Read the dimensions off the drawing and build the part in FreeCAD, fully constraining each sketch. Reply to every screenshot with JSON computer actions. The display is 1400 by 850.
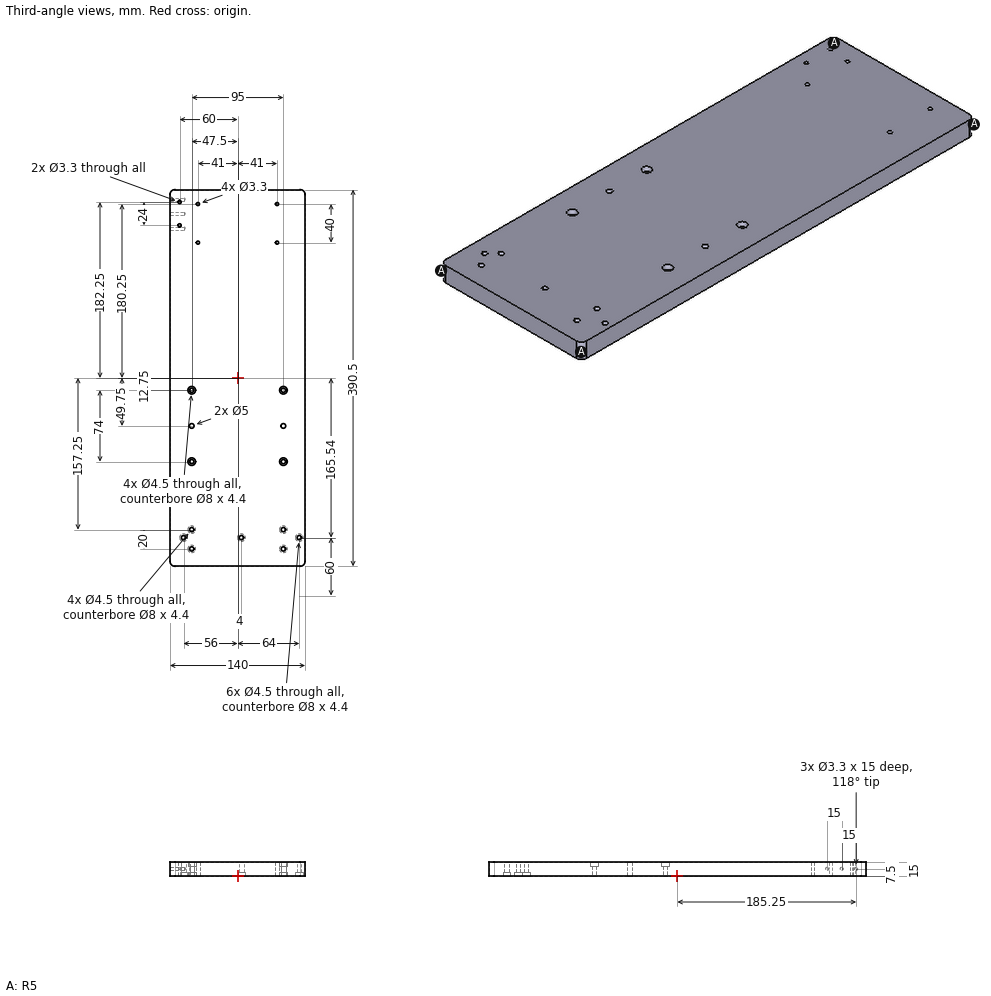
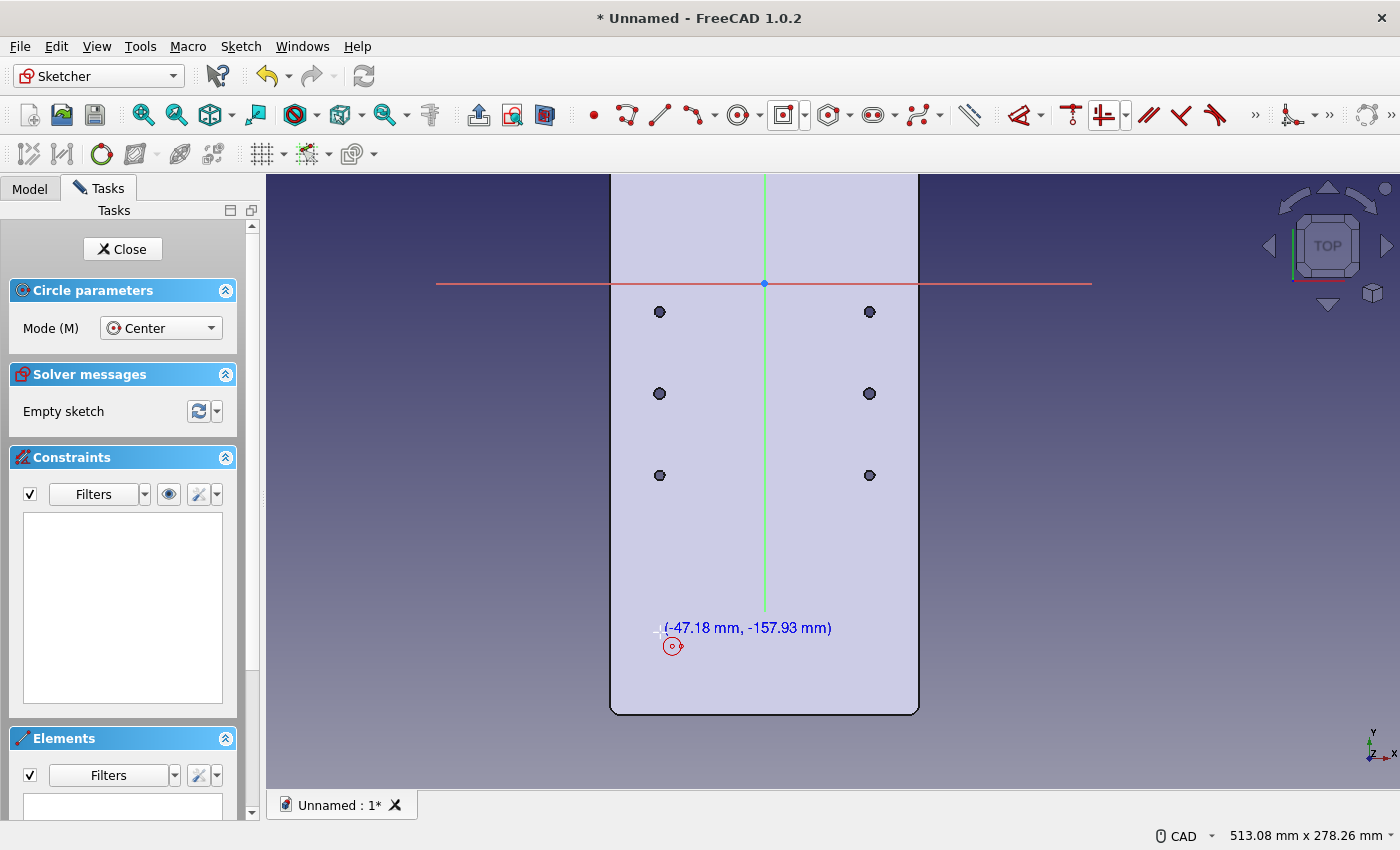
{"action": "left_click", "coordinate": [660, 631]}
{"action": "mouse_move", "coordinate": [663, 628]}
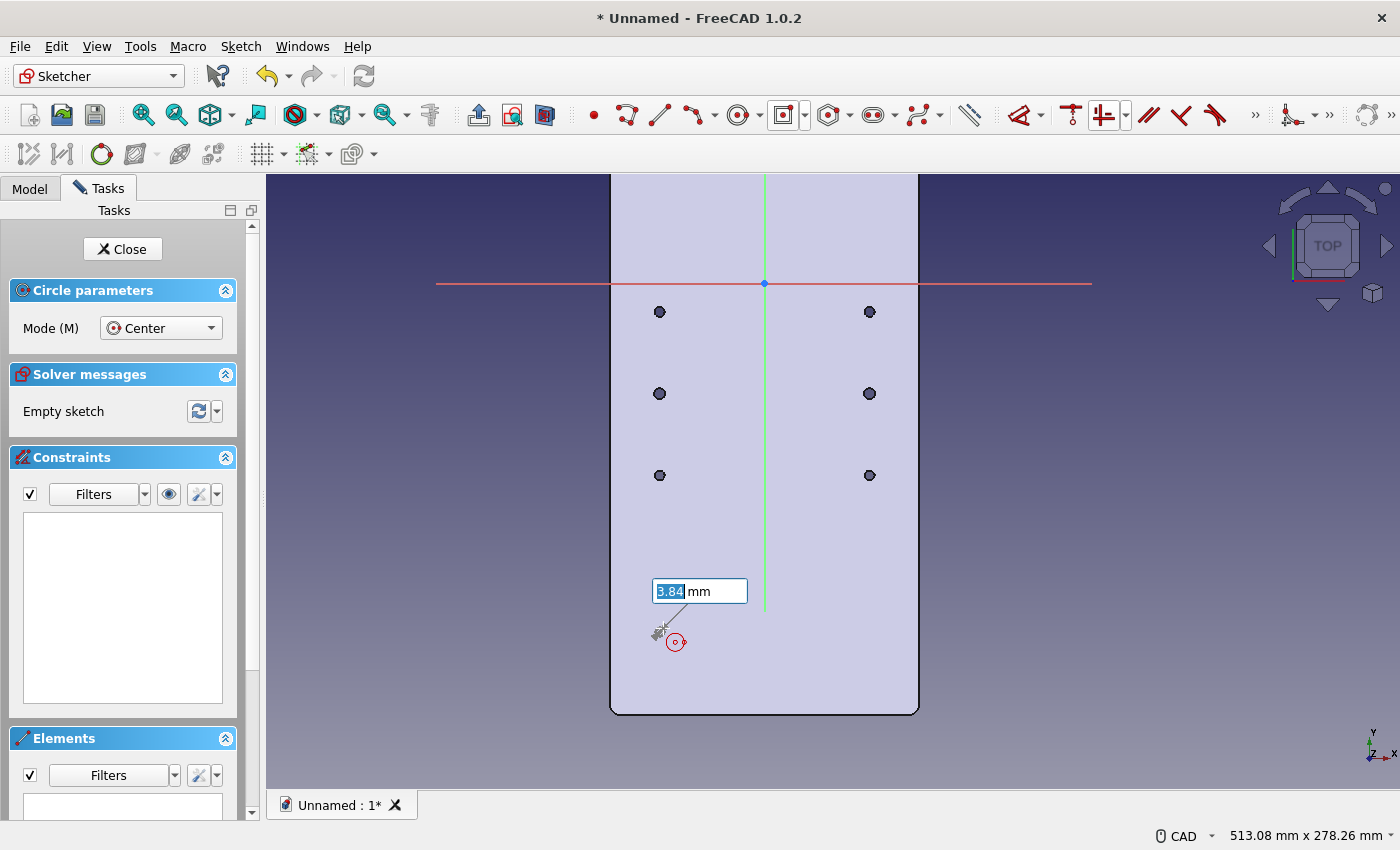
{"action": "type", "text": "4.5"}
{"action": "key", "text": "Return"}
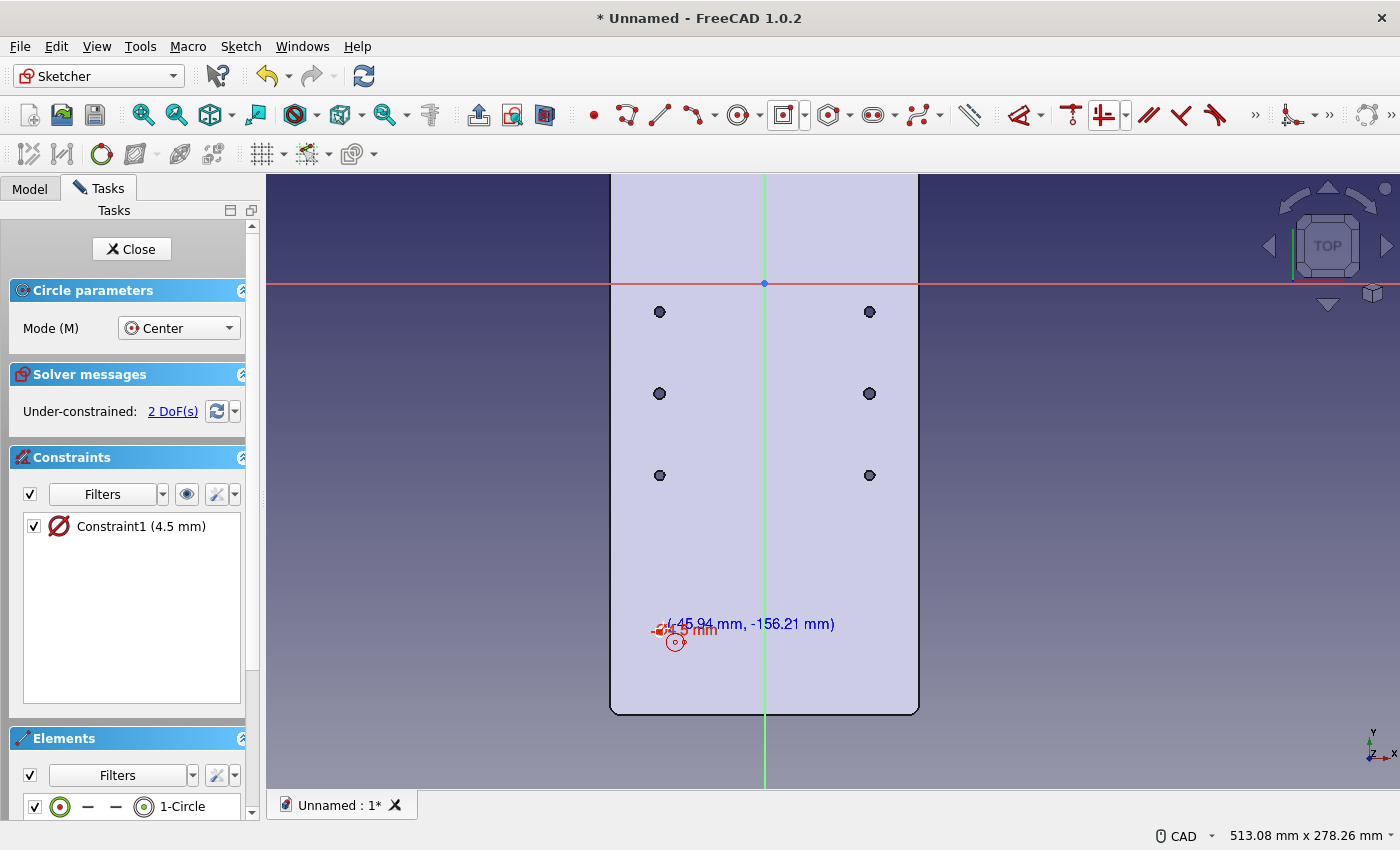
{"action": "scroll", "coordinate": [660, 676], "scroll_direction": "up", "scroll_amount": 8}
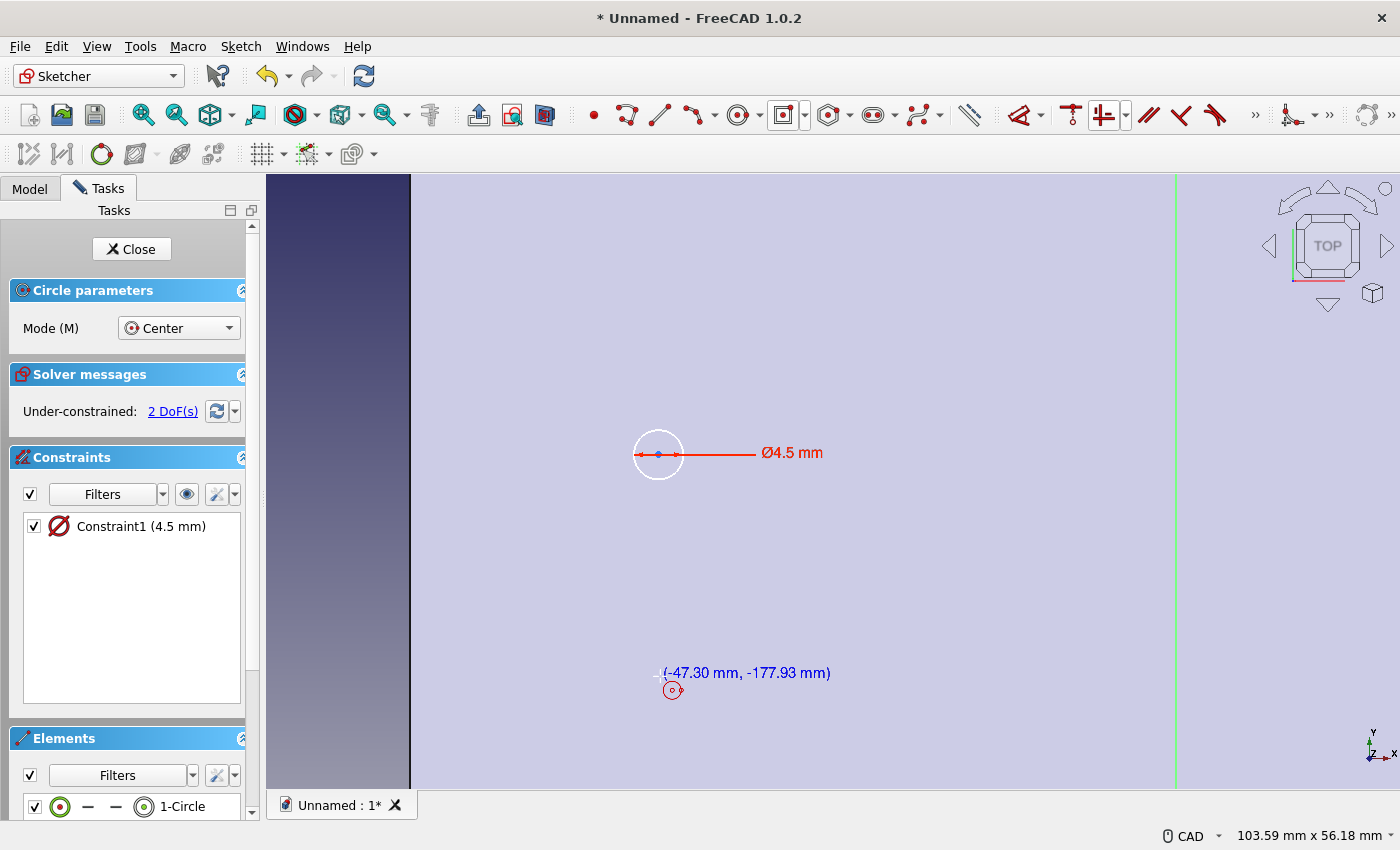
{"action": "scroll", "coordinate": [660, 676], "scroll_direction": "down", "scroll_amount": 8}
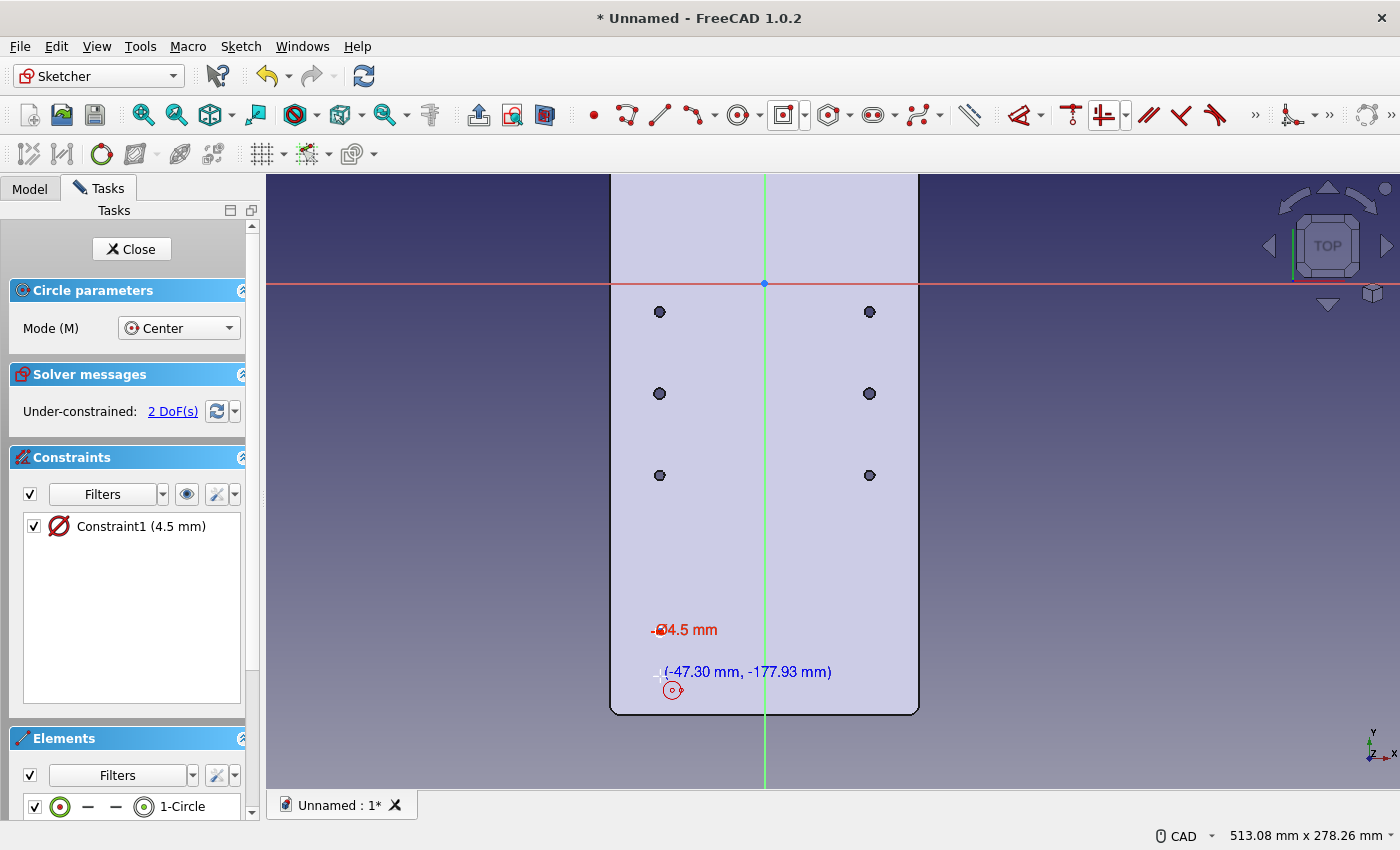
{"action": "left_click", "coordinate": [660, 676]}
{"action": "mouse_move", "coordinate": [663, 672]}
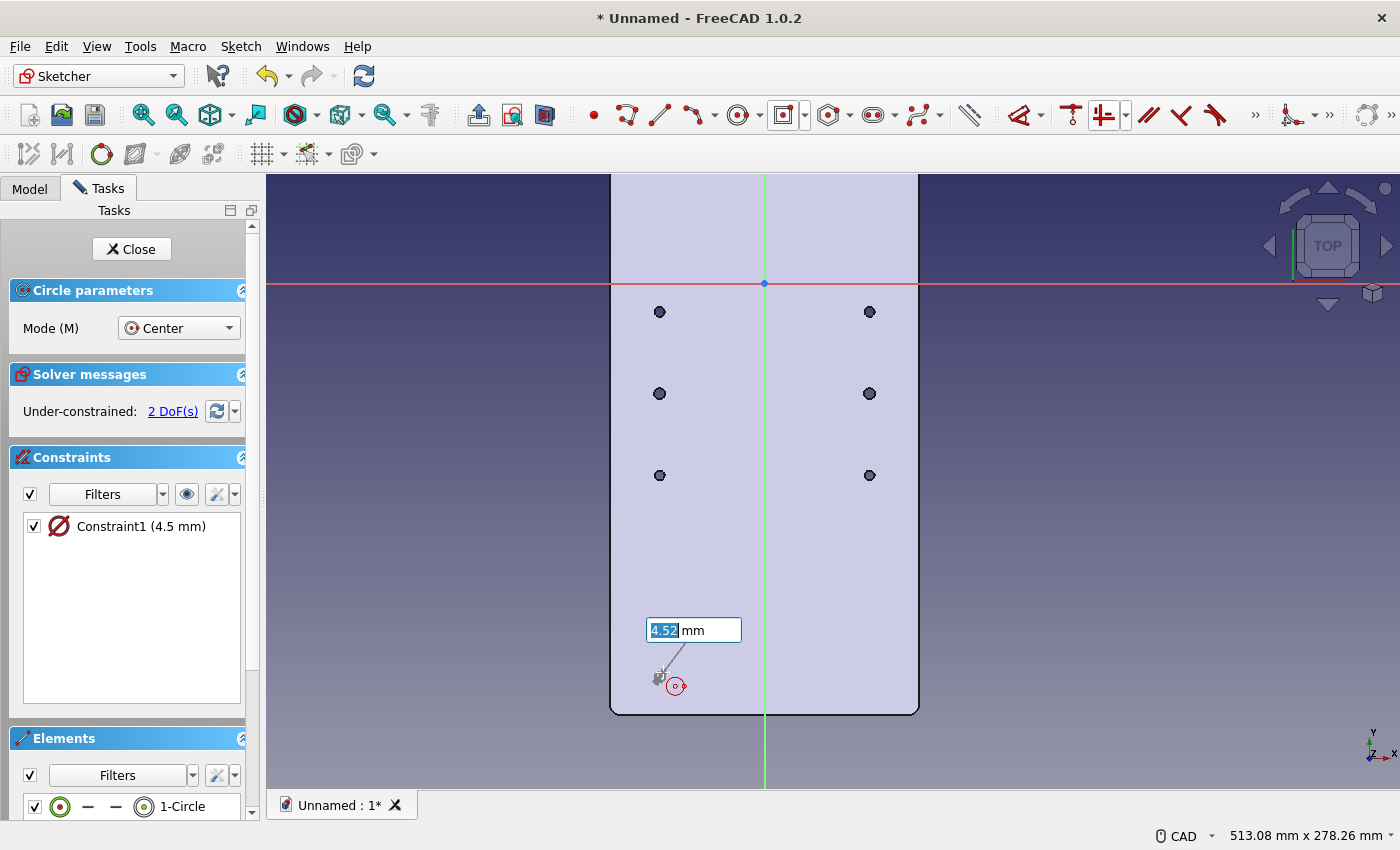
{"action": "type", "text": "4.5"}
{"action": "key", "text": "Return"}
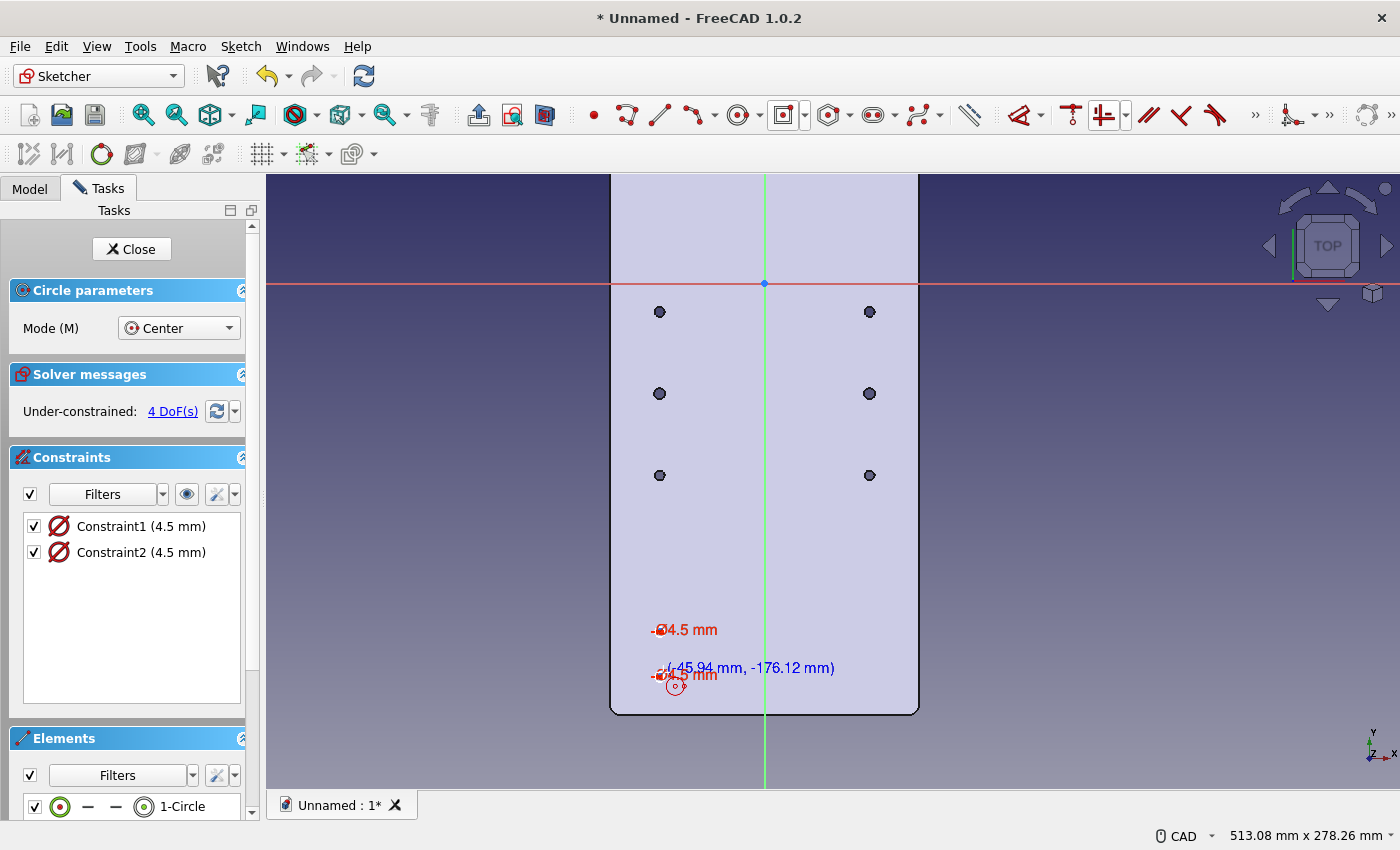
{"action": "scroll", "coordinate": [870, 631], "scroll_direction": "up", "scroll_amount": 8}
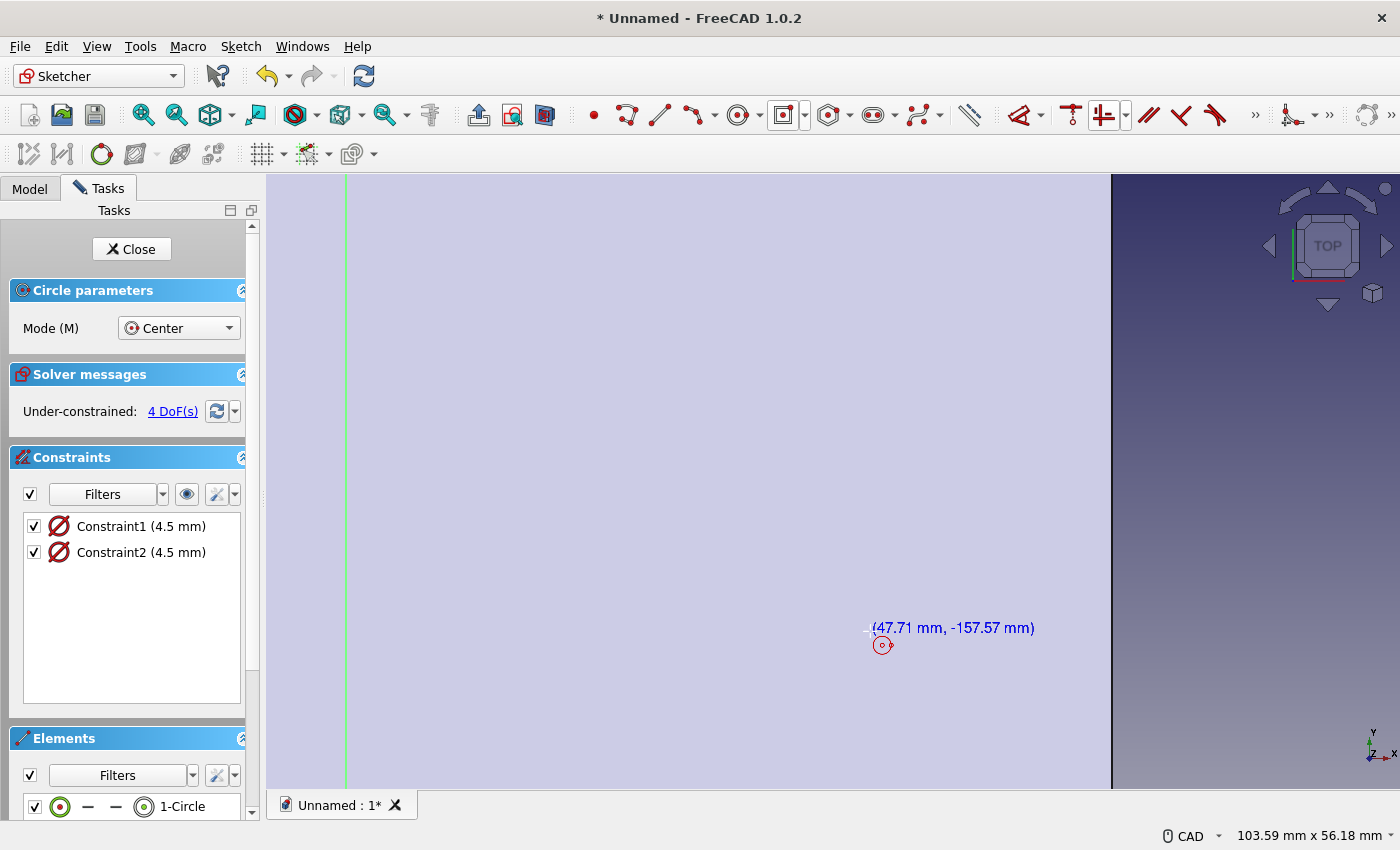
{"action": "scroll", "coordinate": [870, 631], "scroll_direction": "down", "scroll_amount": 8}